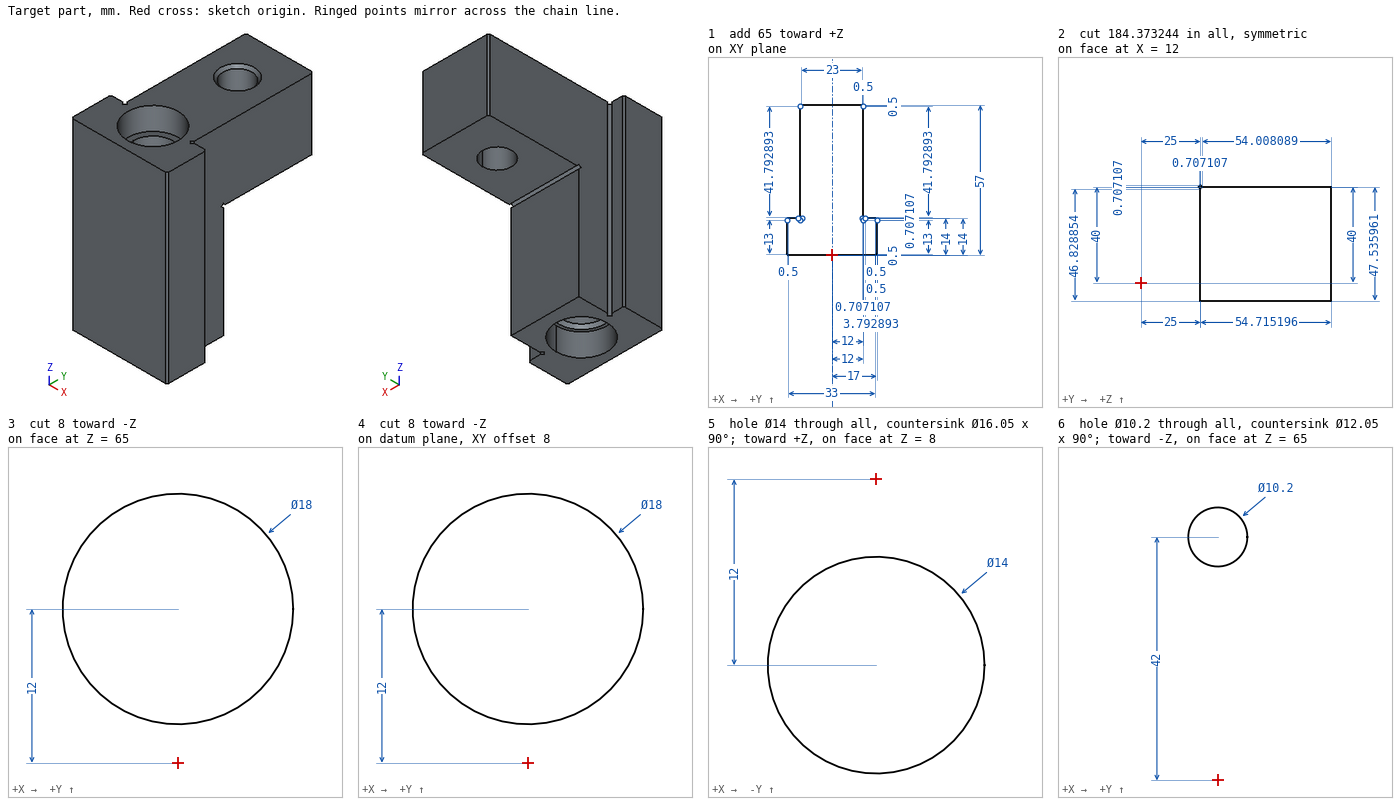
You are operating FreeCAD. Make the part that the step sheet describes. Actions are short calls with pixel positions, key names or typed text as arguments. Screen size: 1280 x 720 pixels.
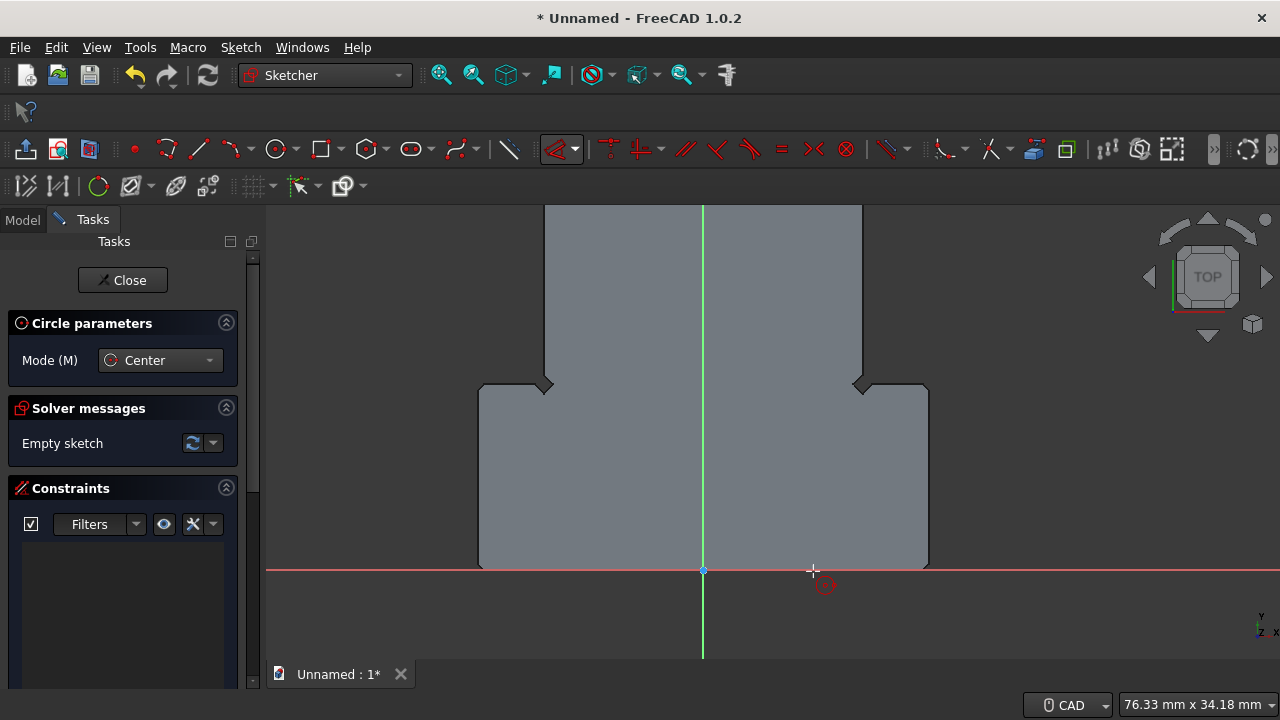
click(703, 411)
click(788, 326)
key(Escape)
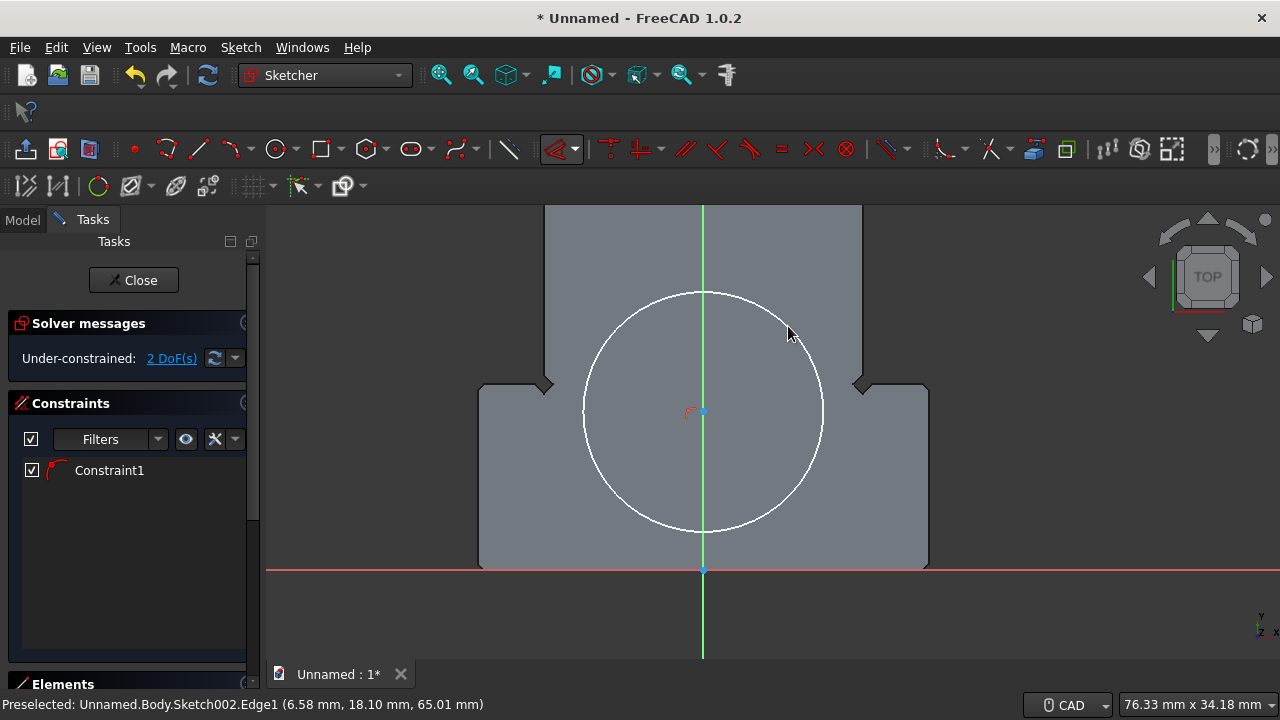
click(556, 150)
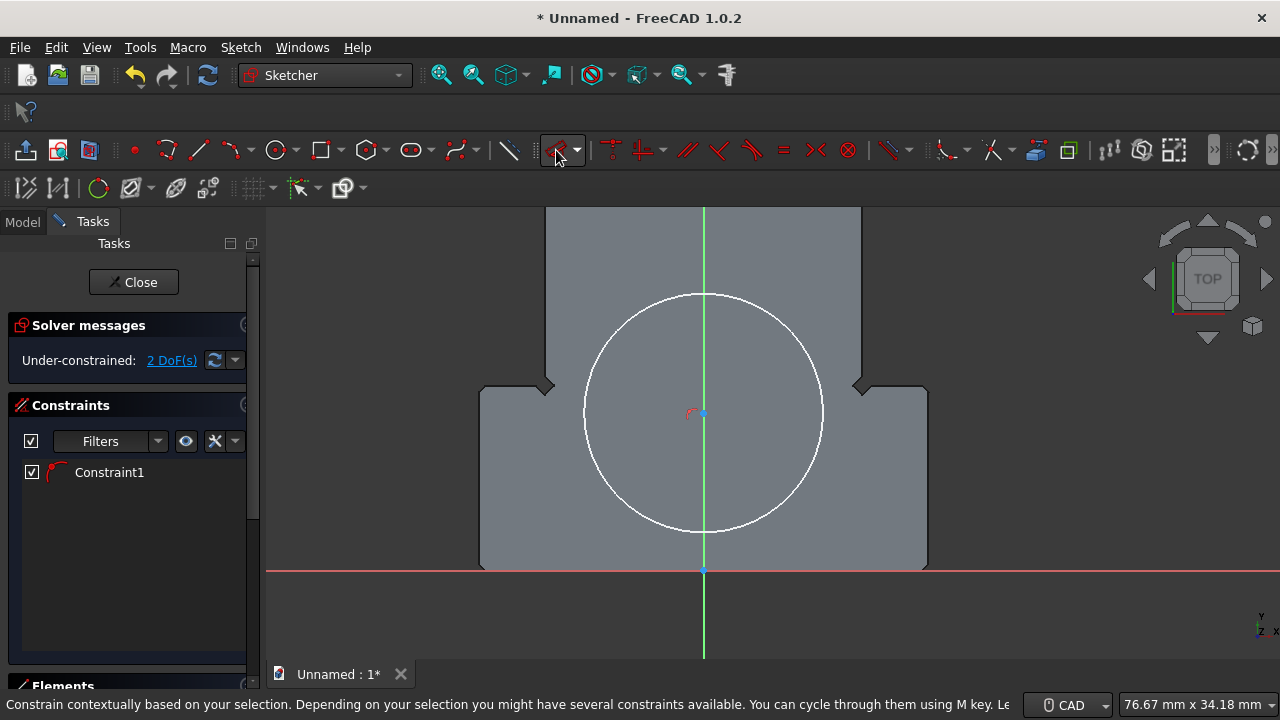
click(788, 328)
click(811, 305)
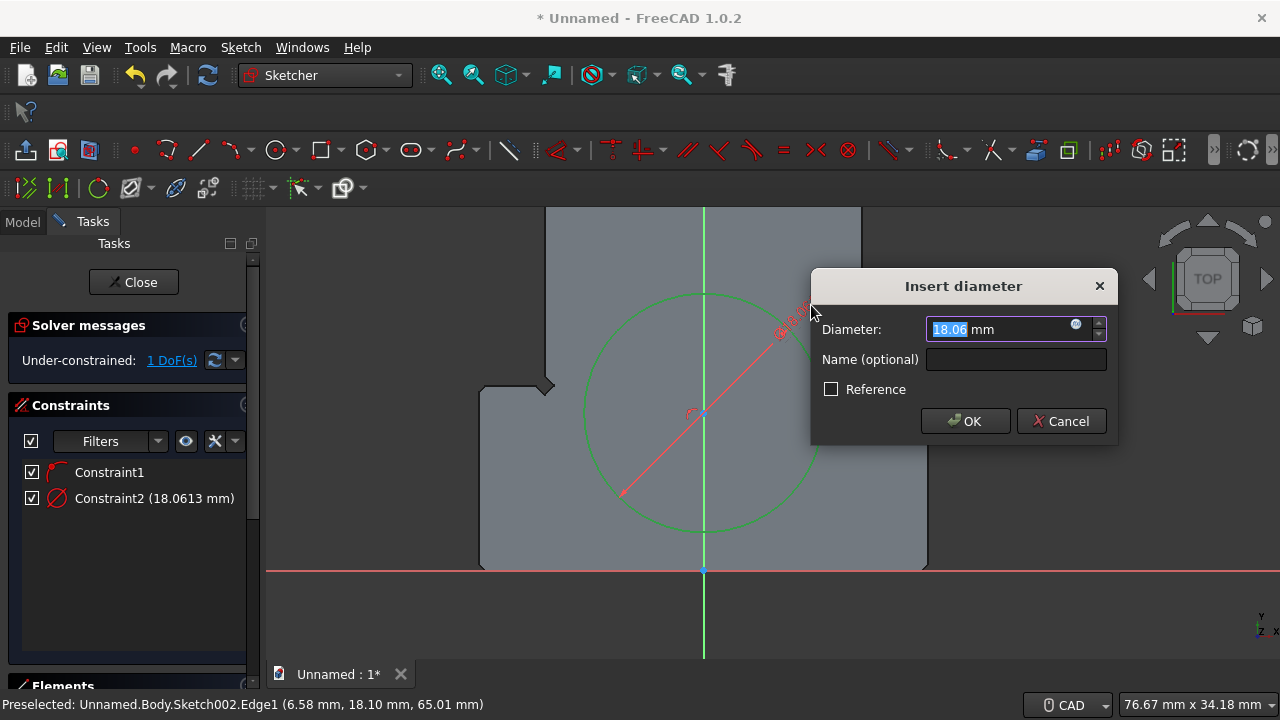
text(18)
key(Return)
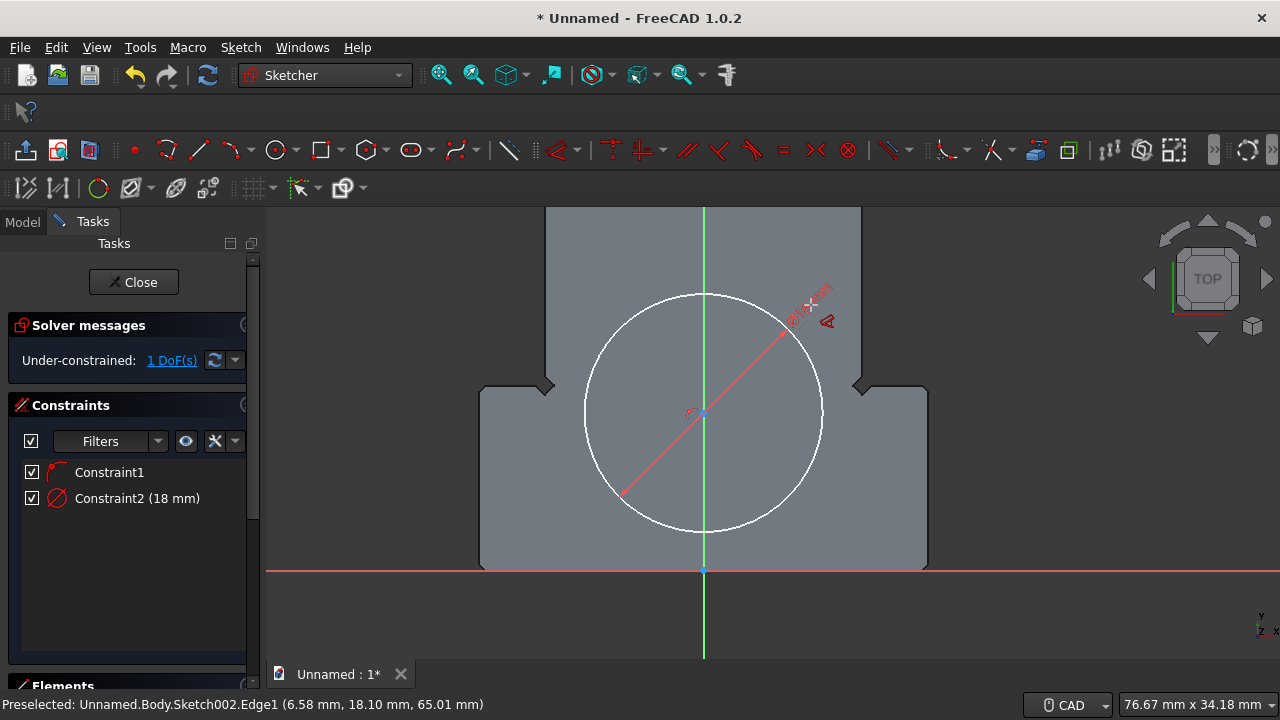
click(704, 413)
click(738, 492)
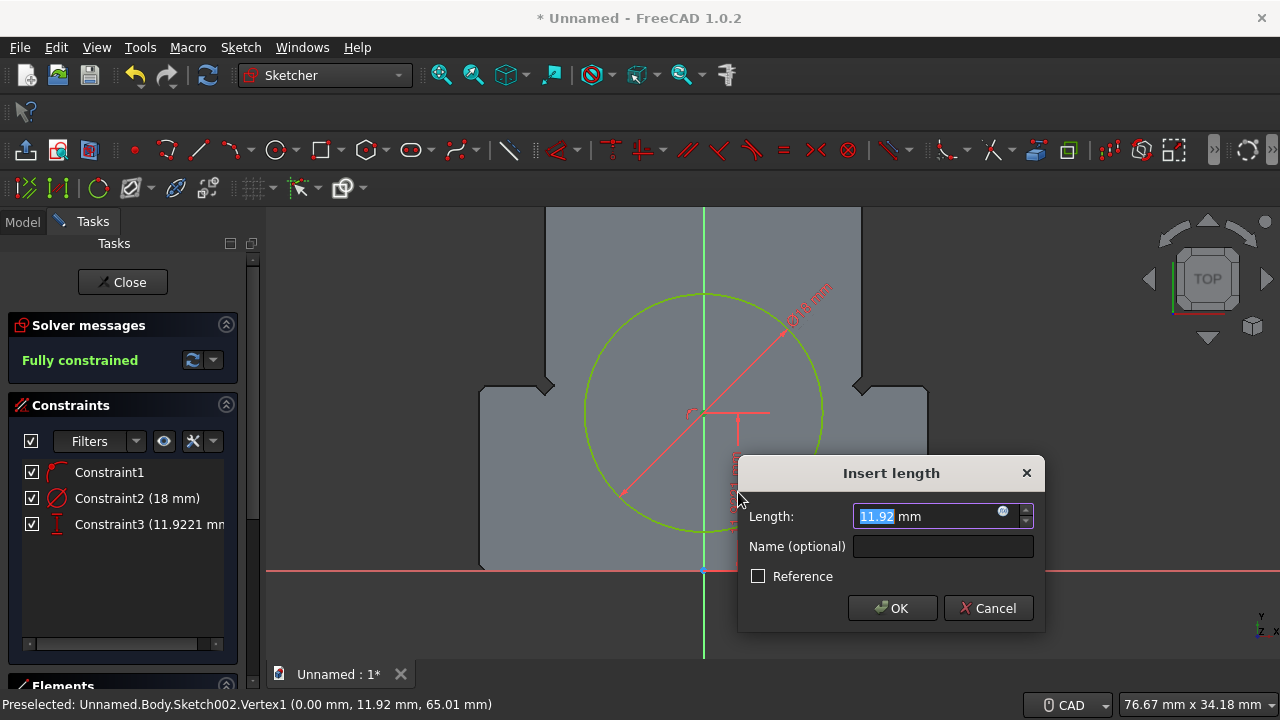
text(12)
key(Return)
key(Escape)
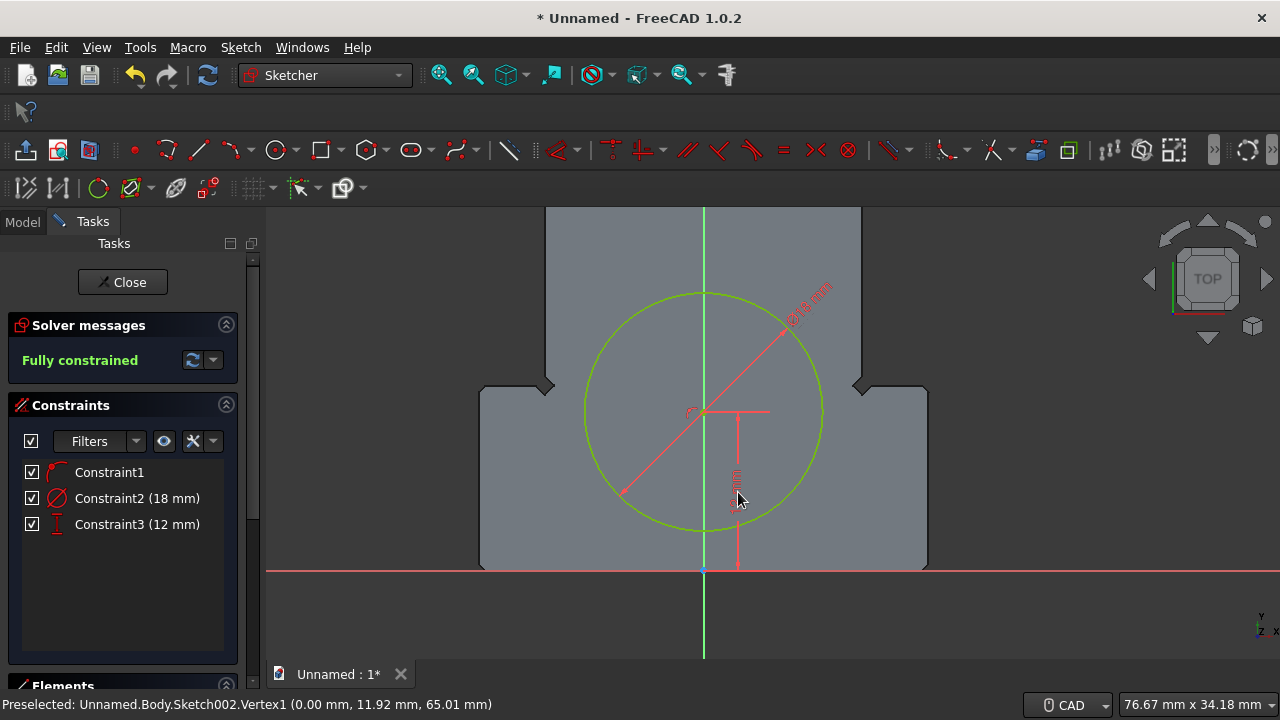
click(123, 282)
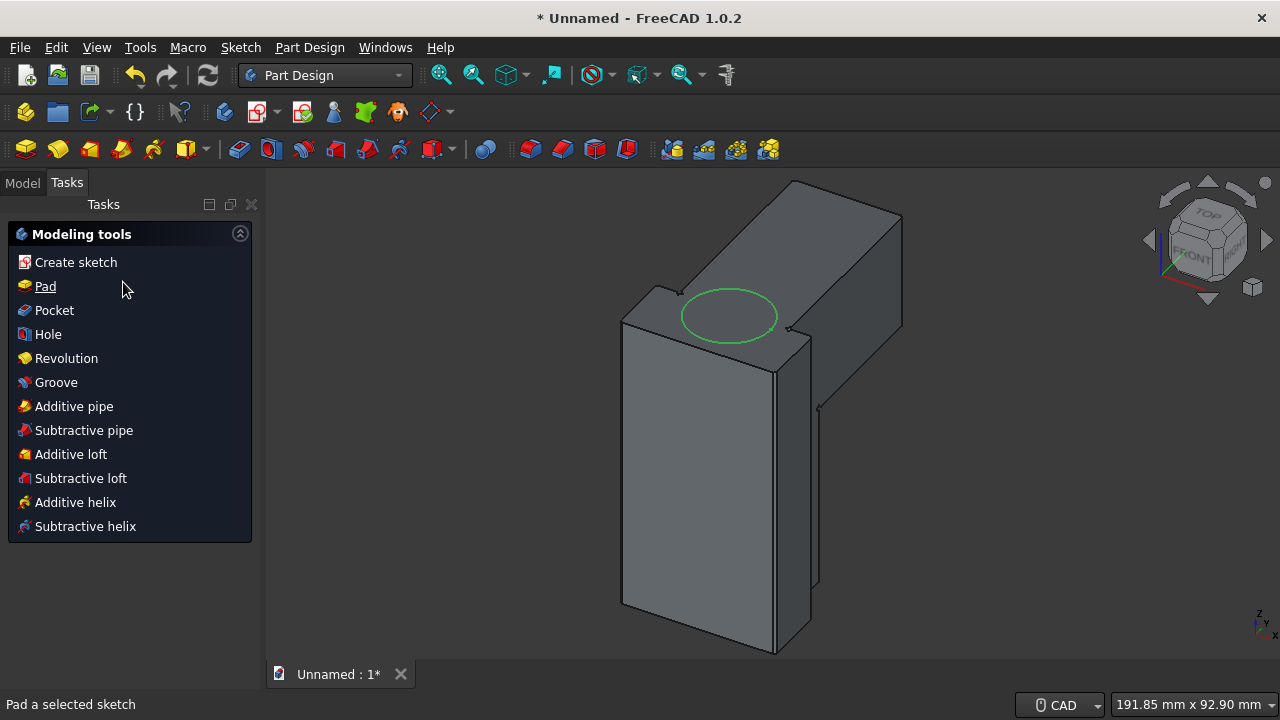
click(240, 150)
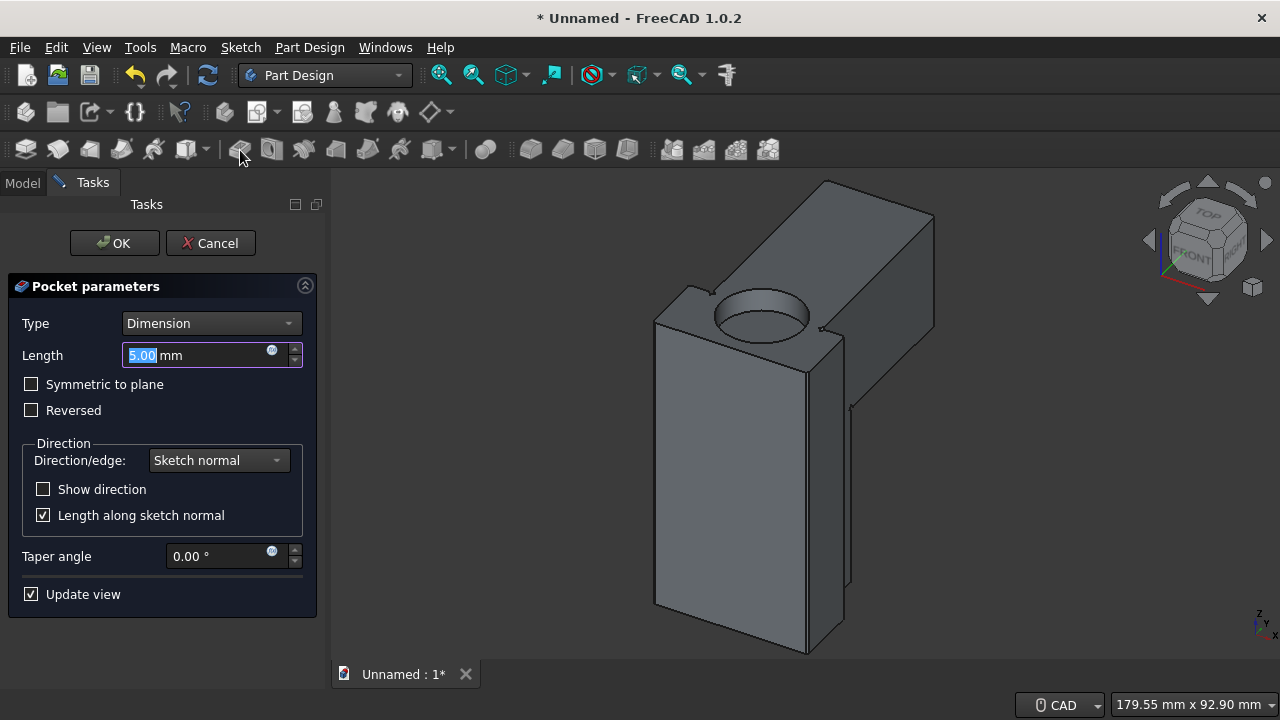
text(8)
key(Tab)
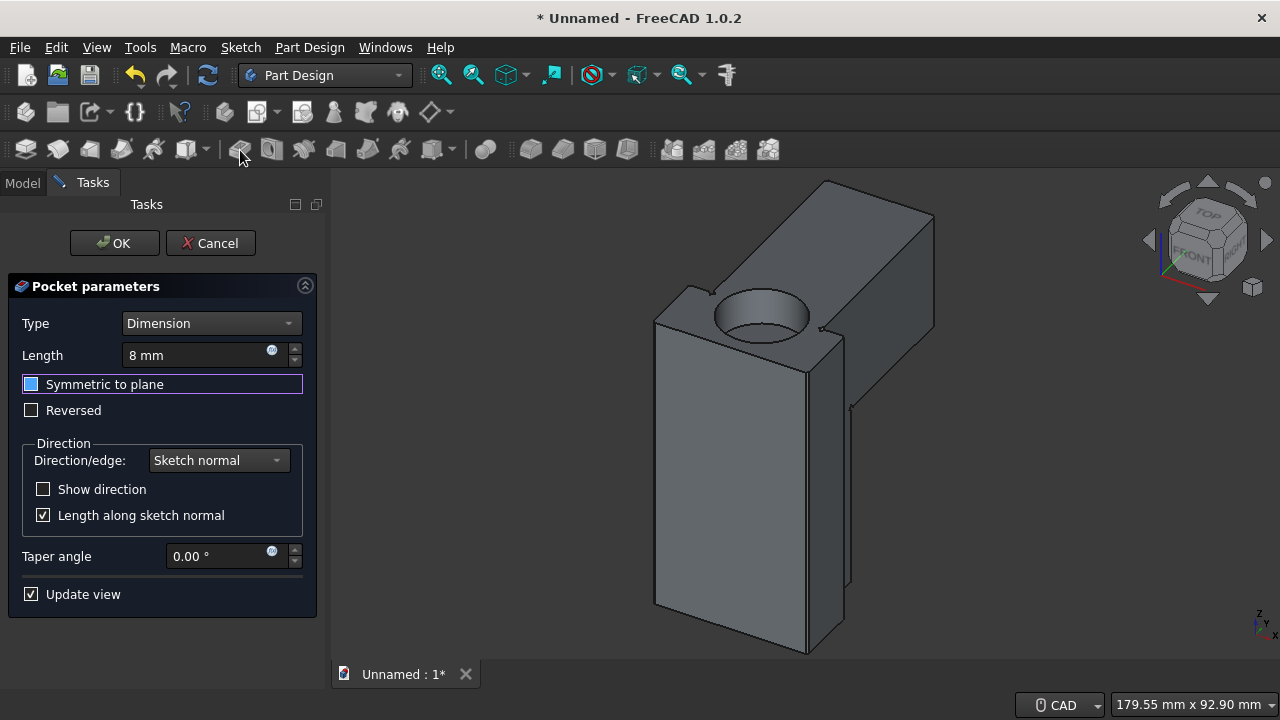
click(115, 243)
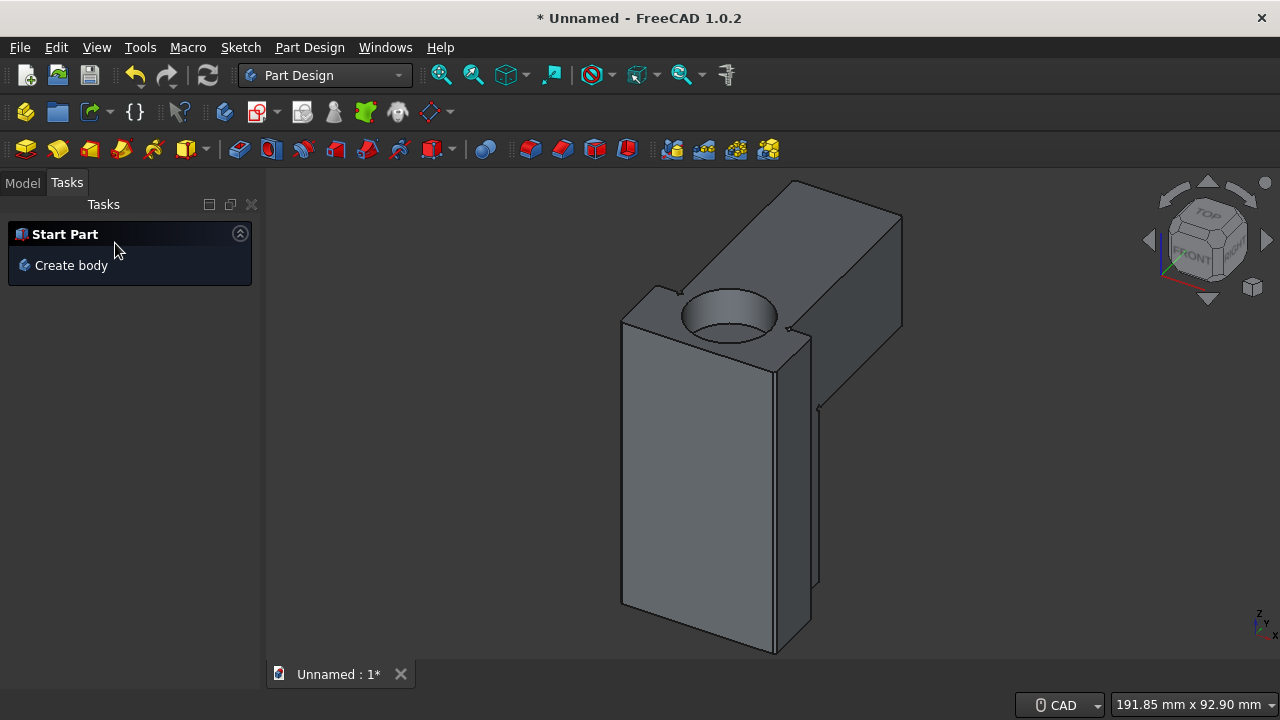
click(23, 182)